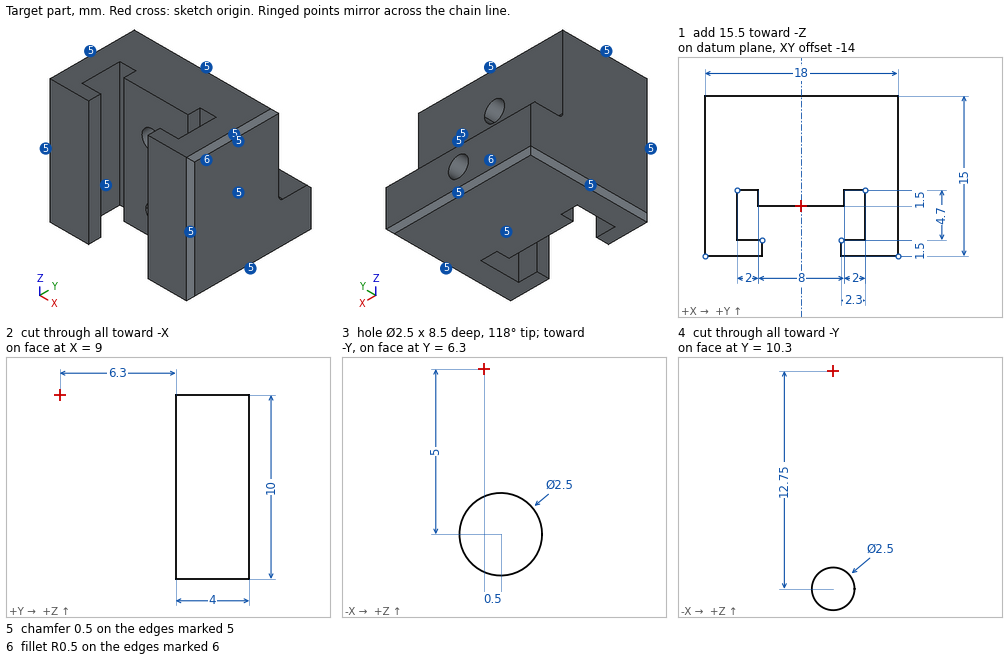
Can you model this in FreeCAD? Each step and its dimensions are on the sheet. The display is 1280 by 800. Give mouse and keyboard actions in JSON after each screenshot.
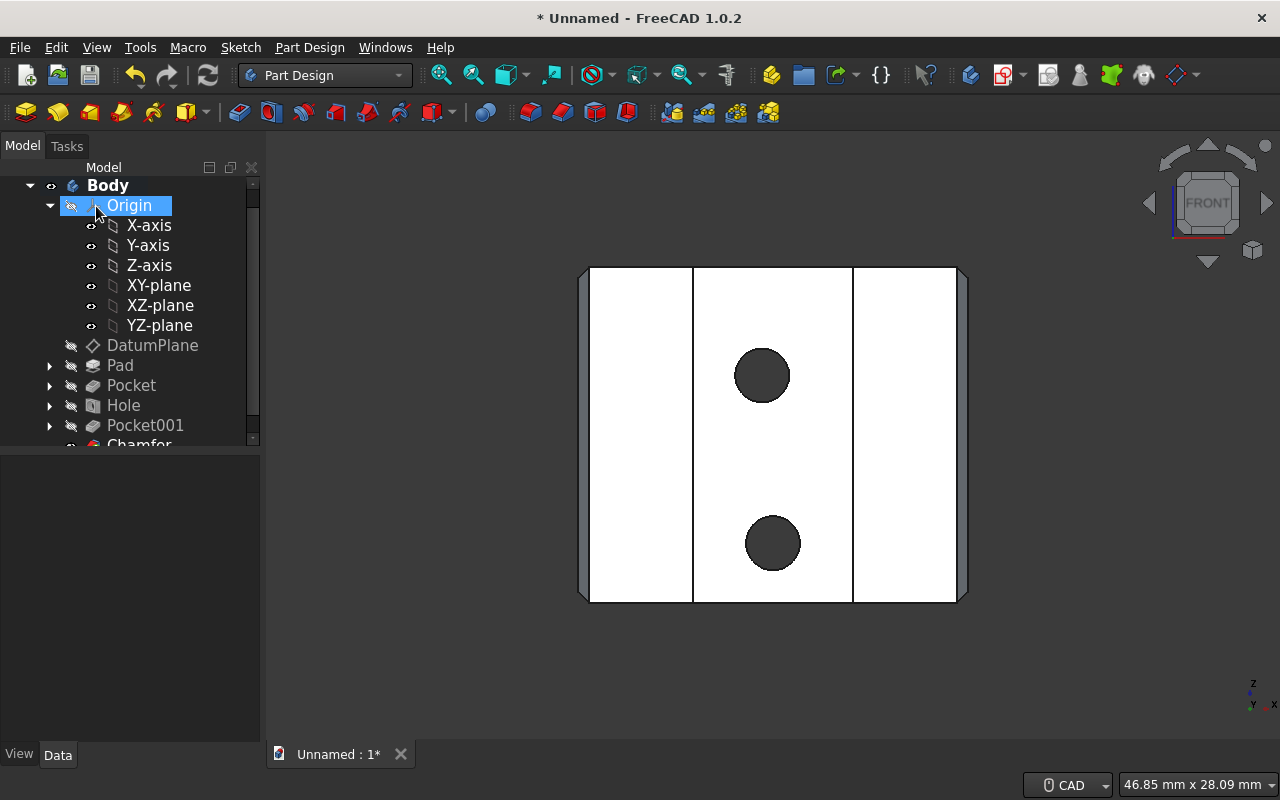
{"action": "key", "text": "3"}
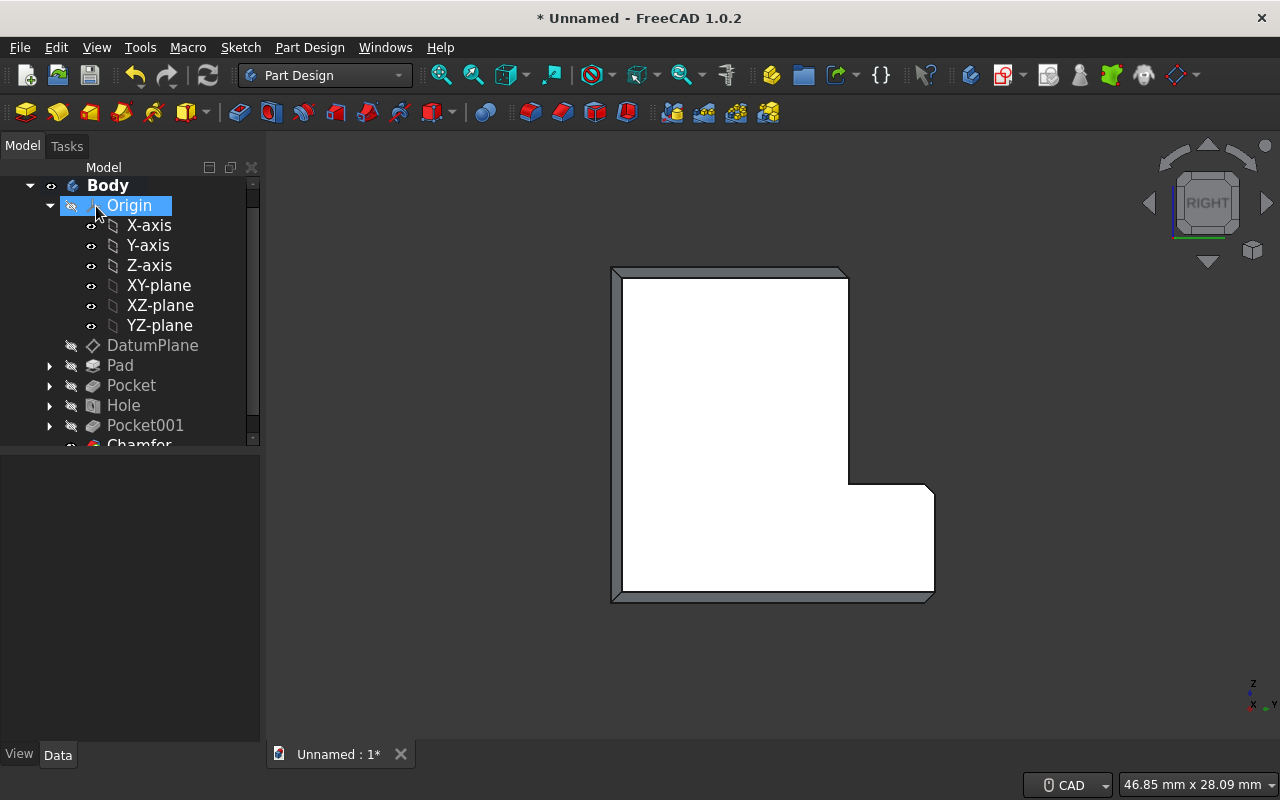
{"action": "key", "text": "5"}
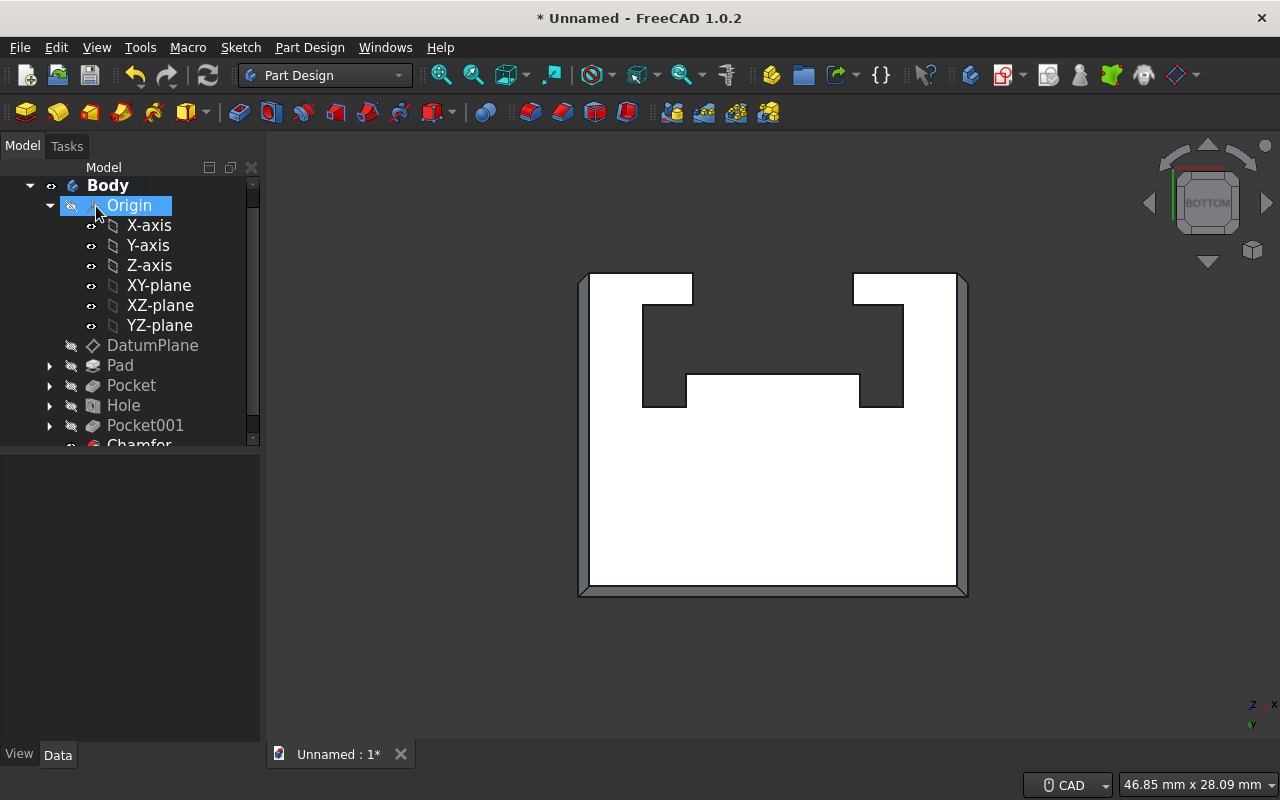
{"action": "key", "text": "4"}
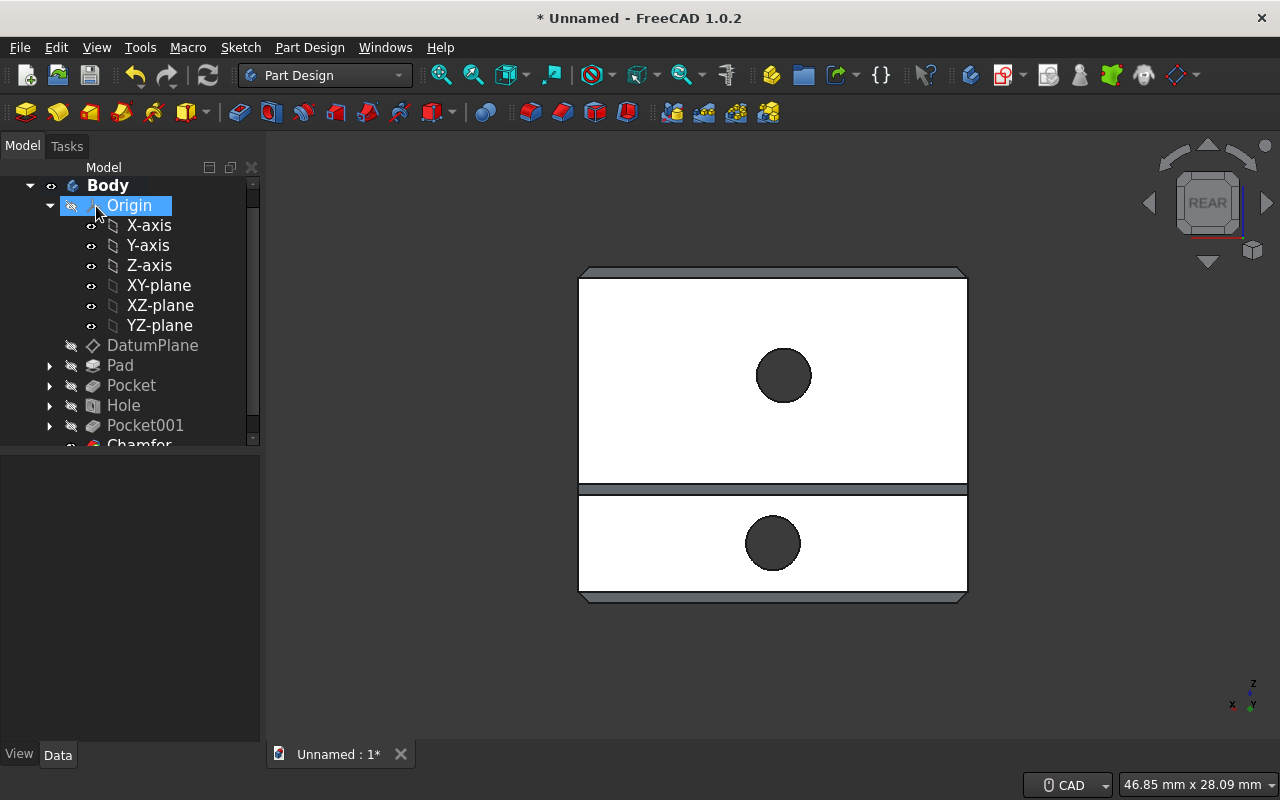
{"action": "key", "text": "6"}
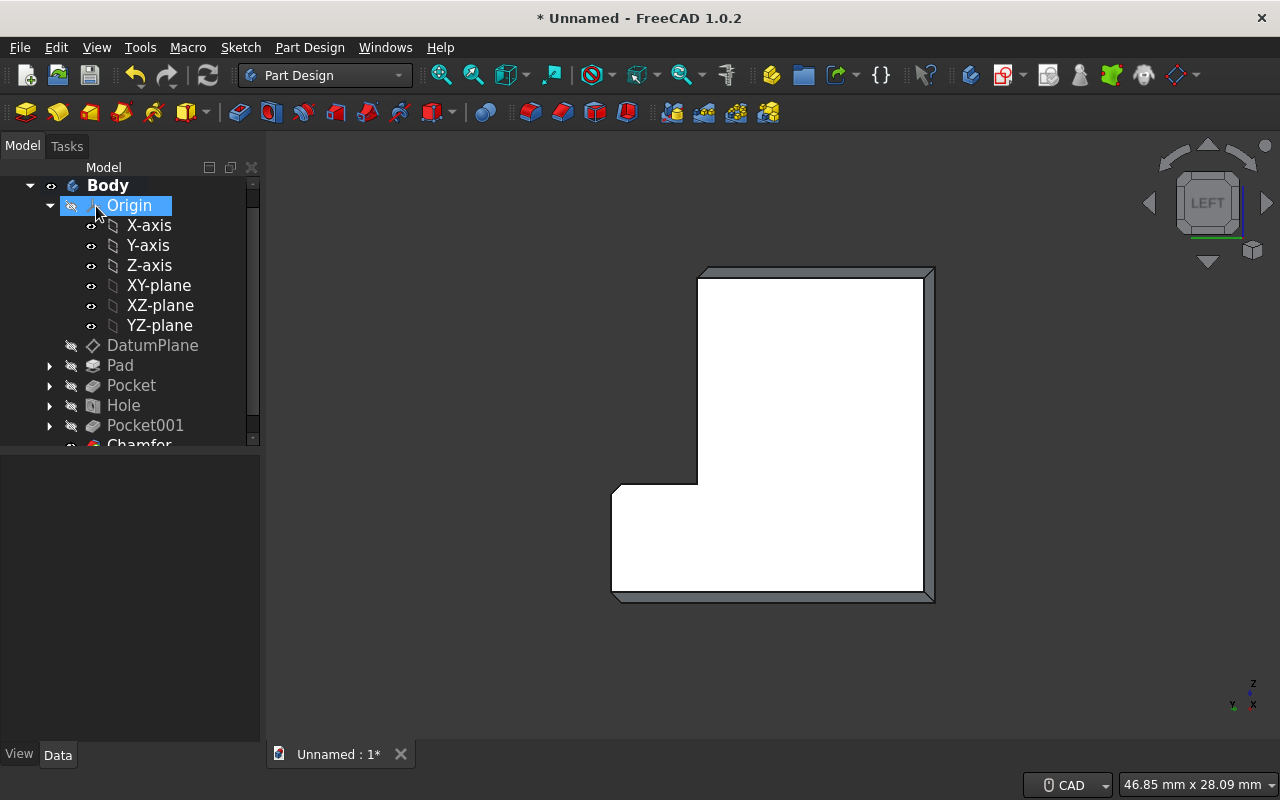
{"action": "key", "text": "v 3"}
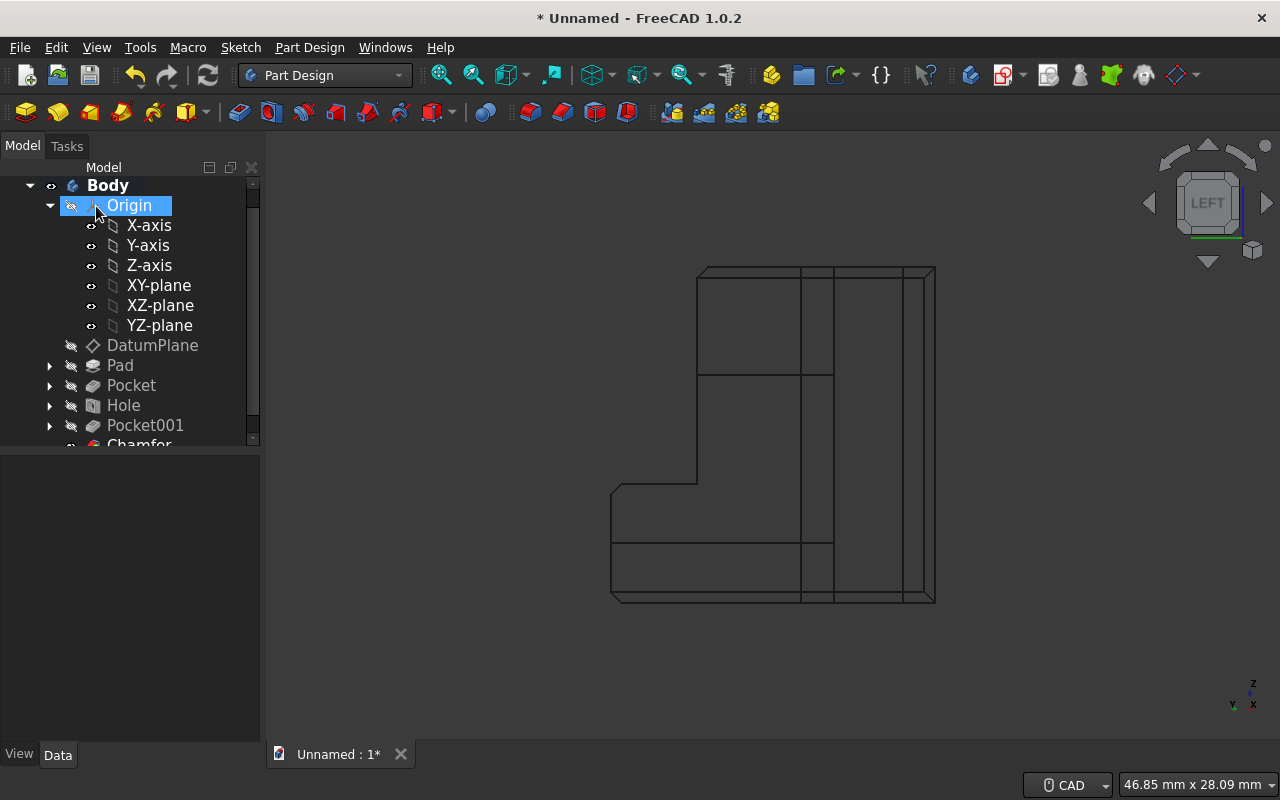
{"action": "key", "text": "0"}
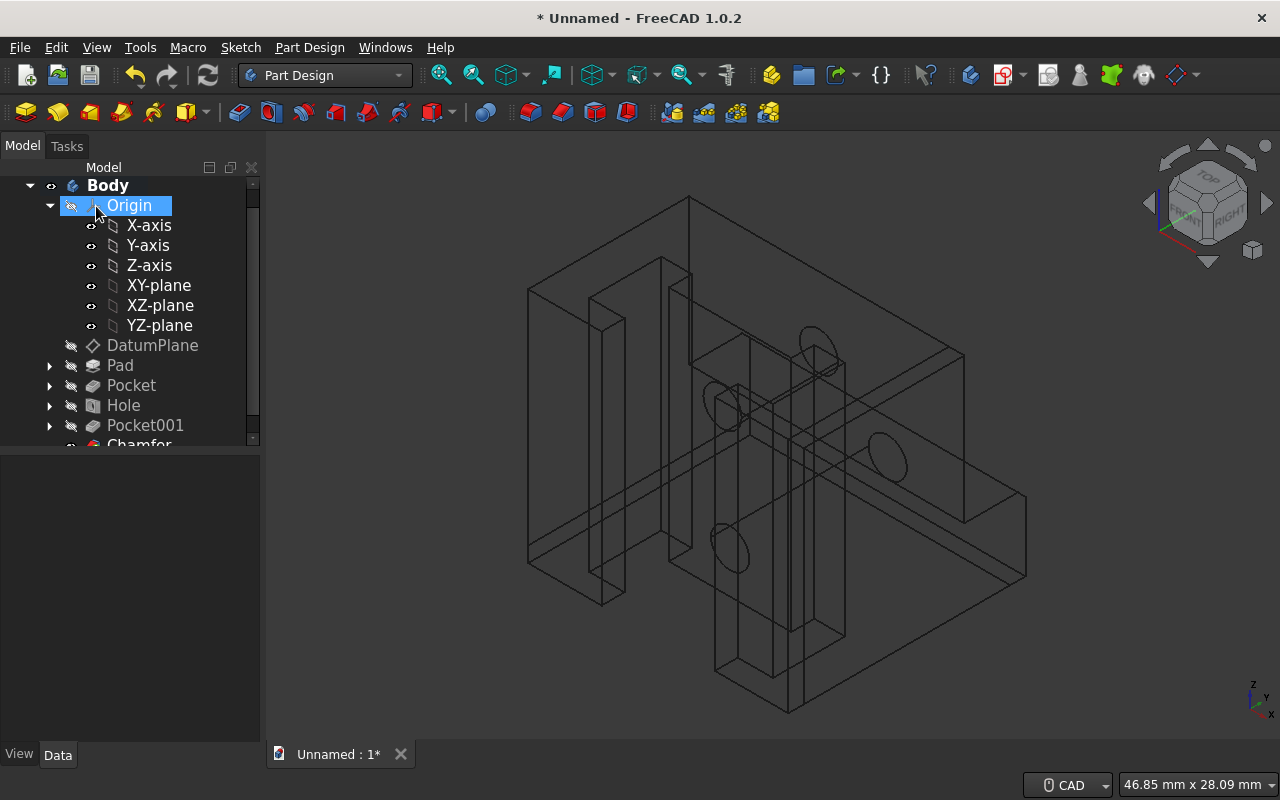
{"action": "left_click", "coordinate": [827, 443]}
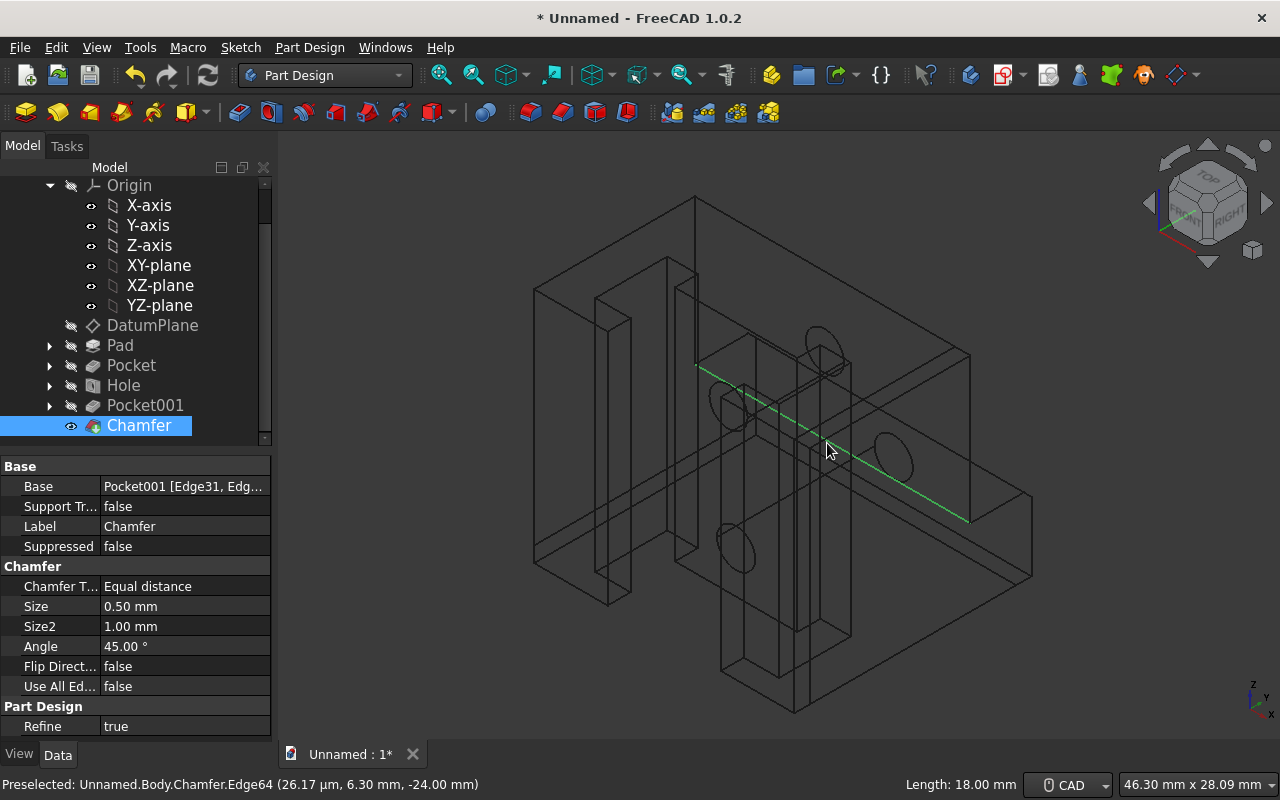
{"action": "key", "text": "v 1"}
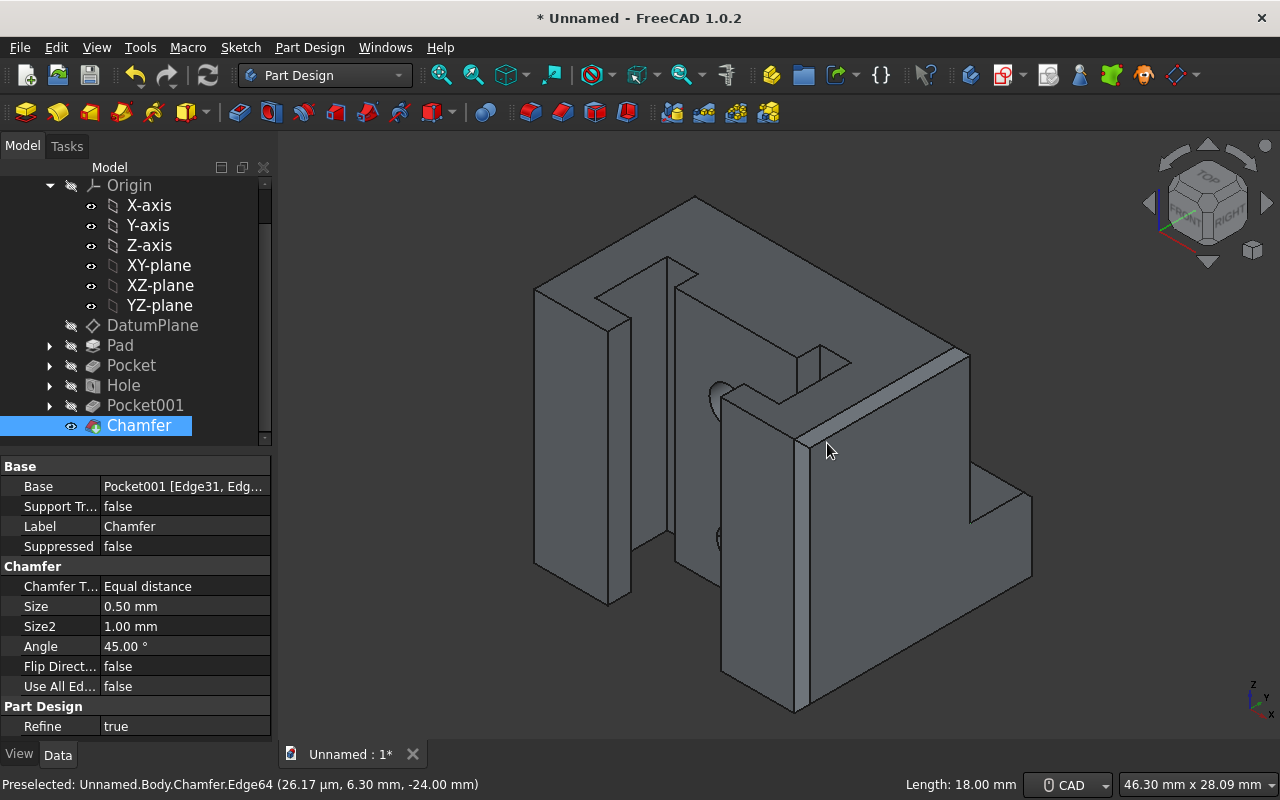
{"action": "left_click", "coordinate": [532, 112]}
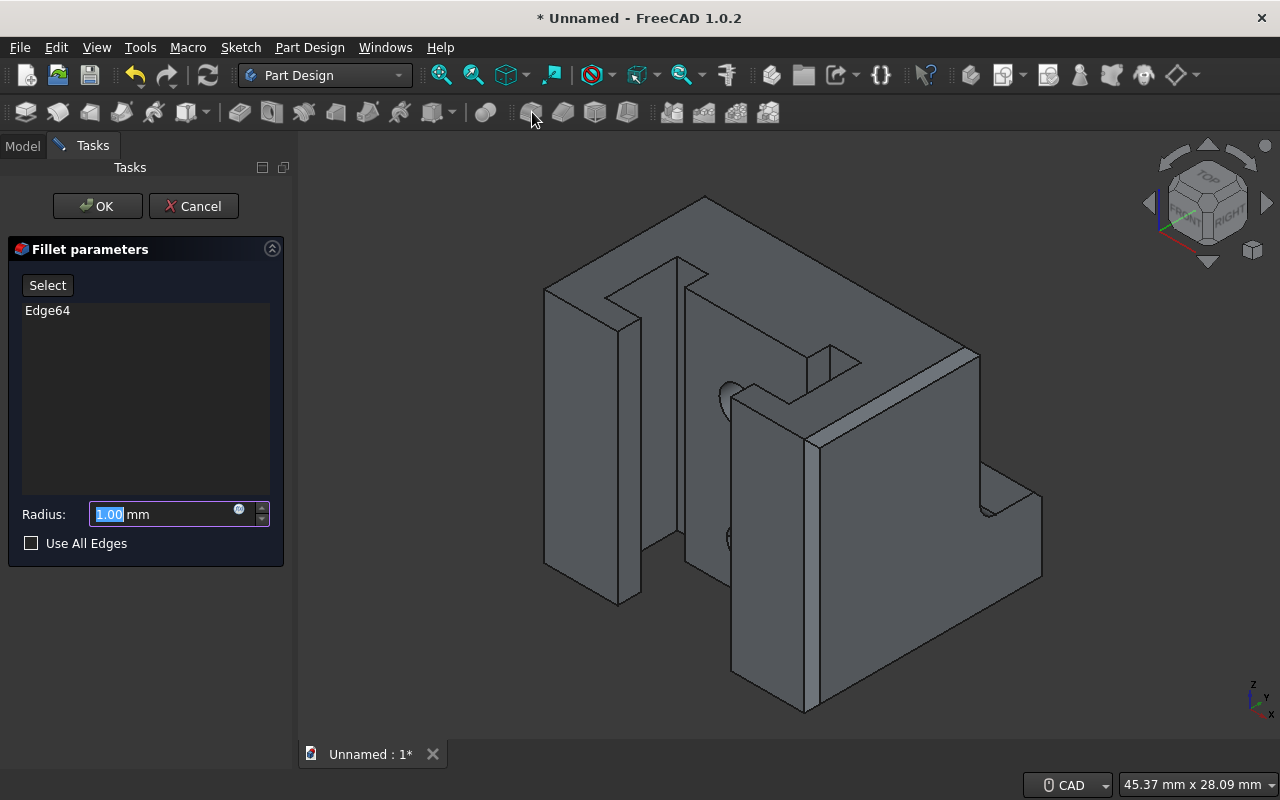
{"action": "type", "text": "0.5"}
{"action": "key", "text": "Tab"}